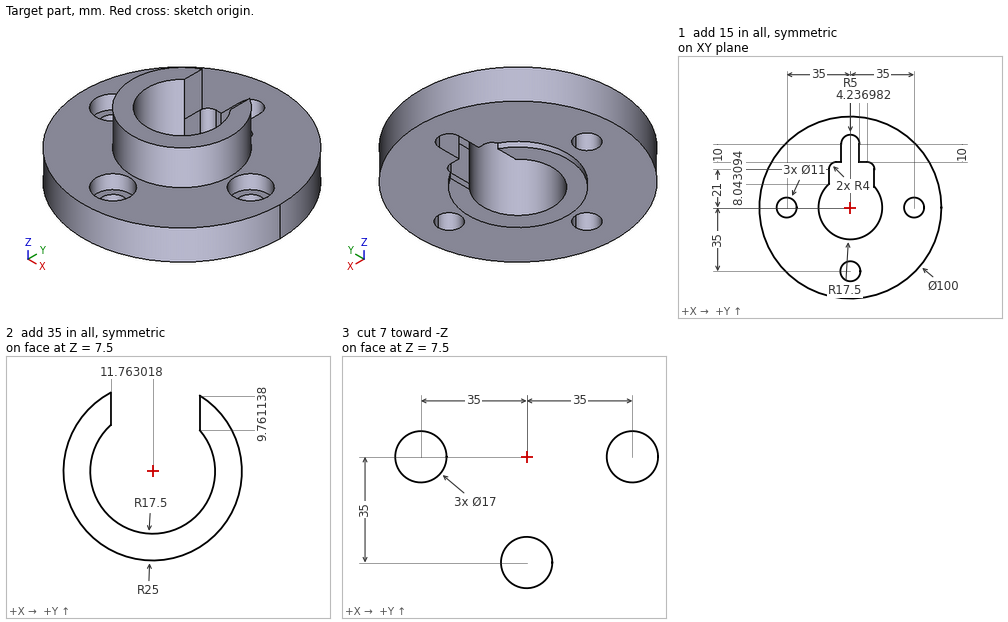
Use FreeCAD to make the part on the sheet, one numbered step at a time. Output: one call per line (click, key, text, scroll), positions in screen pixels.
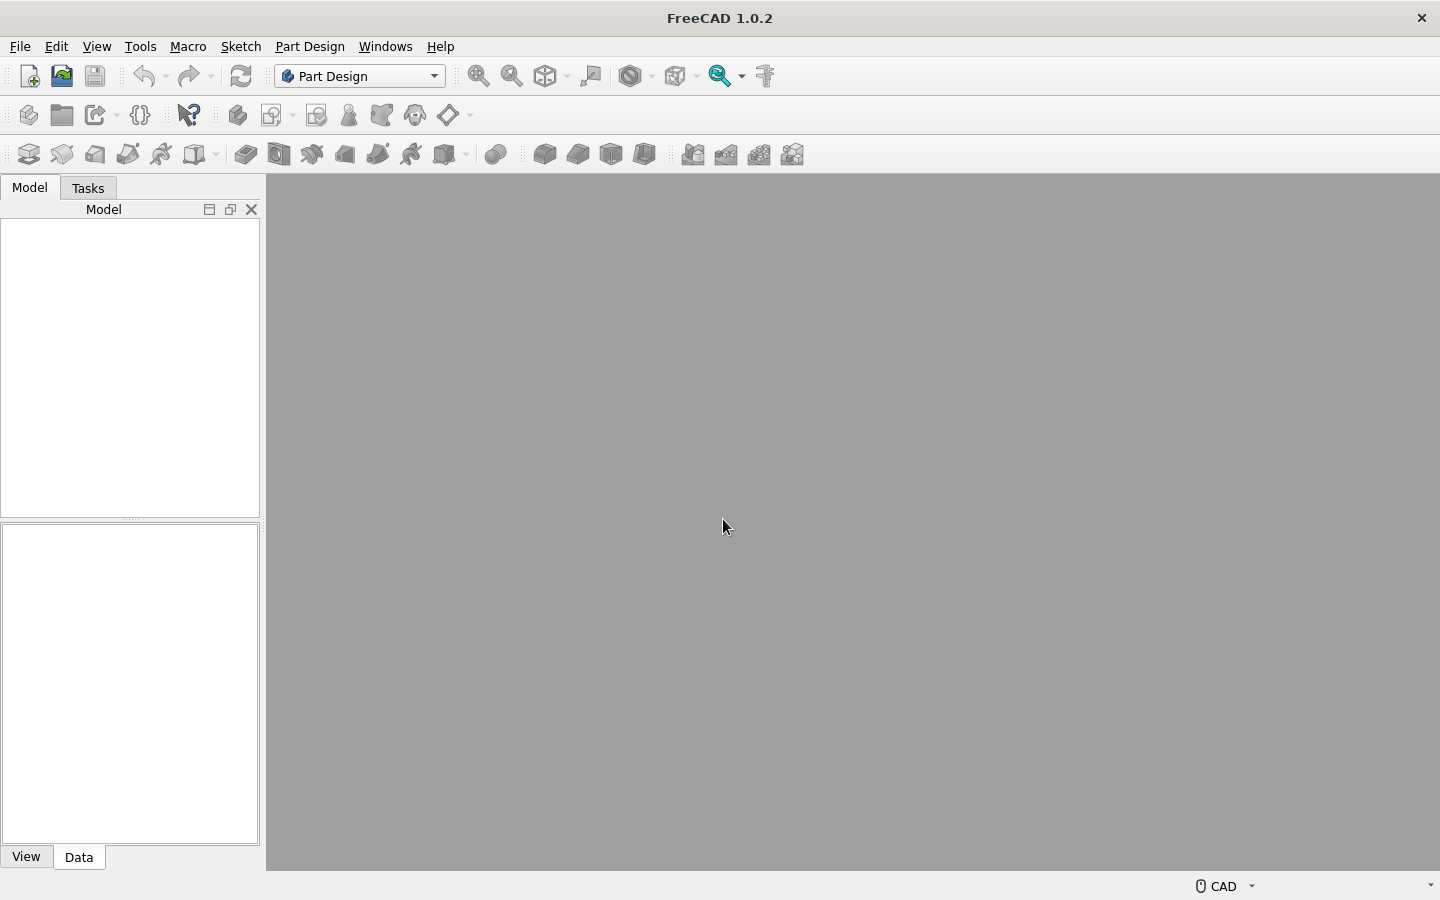
click(29, 76)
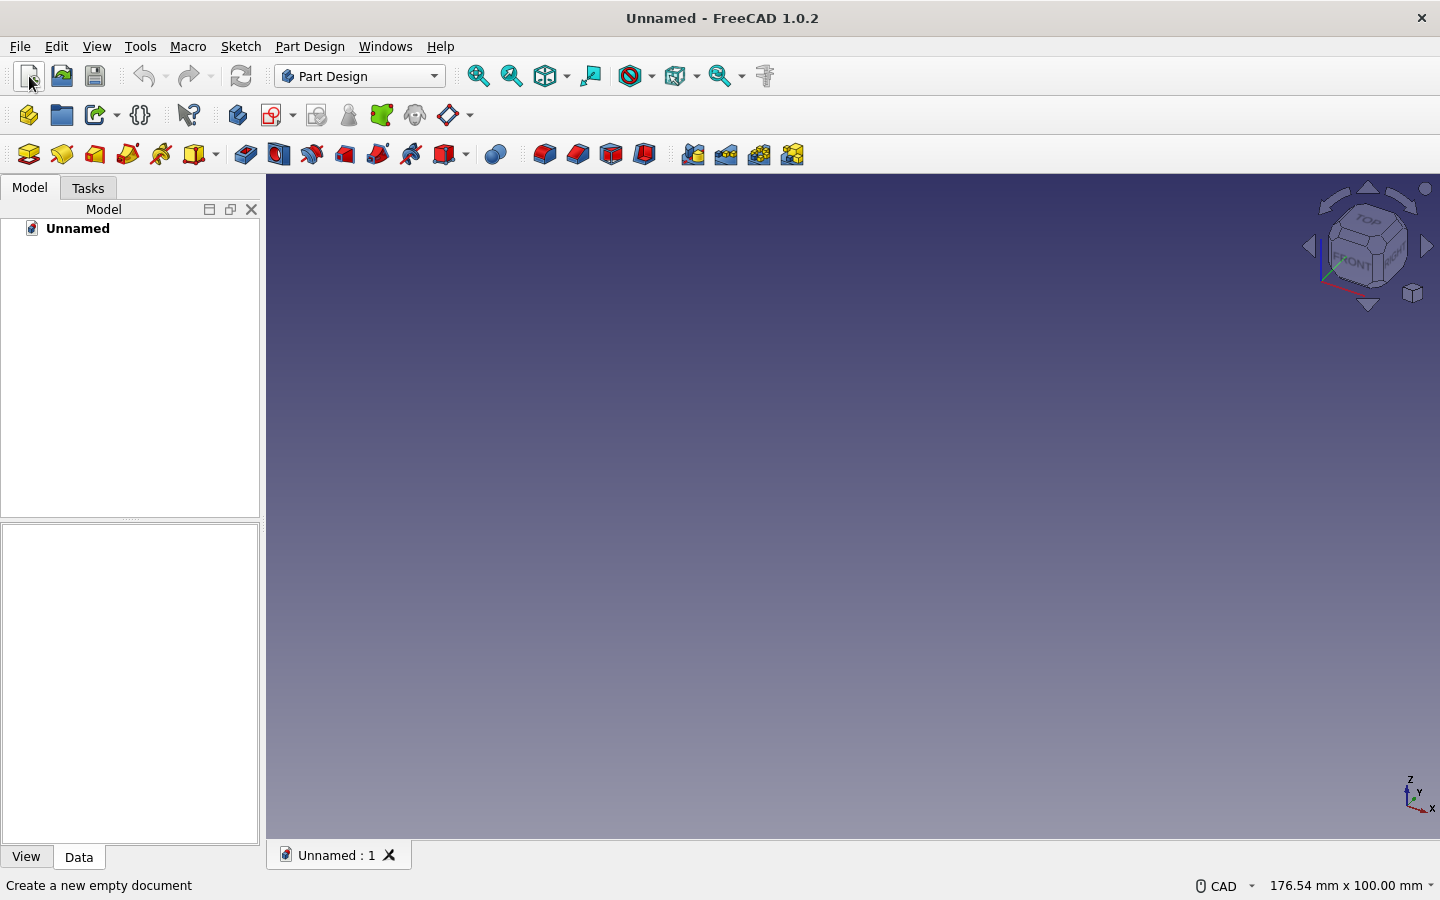
click(270, 116)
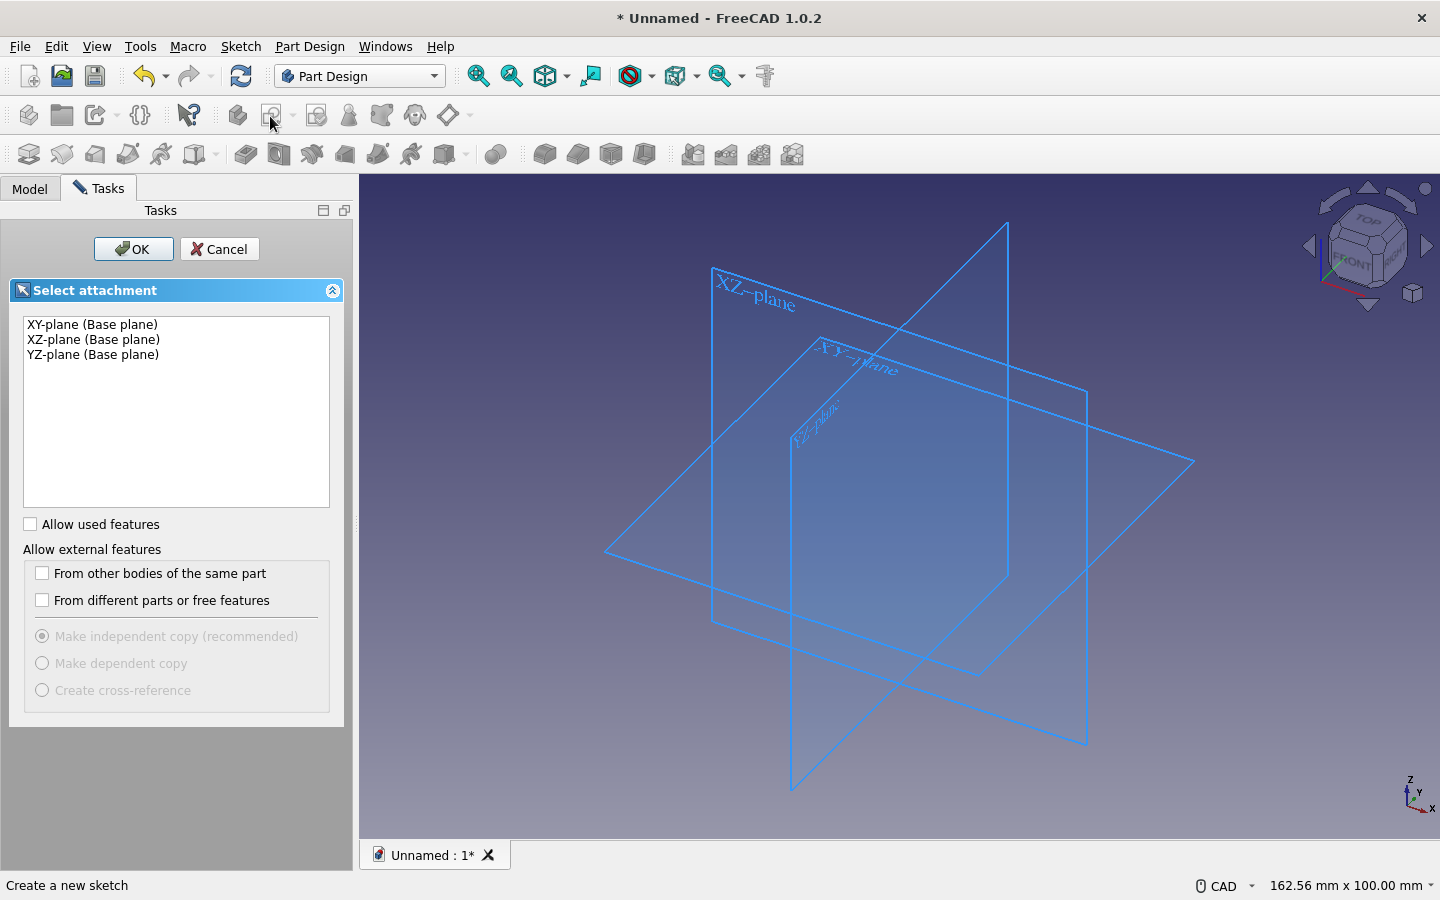
click(84, 324)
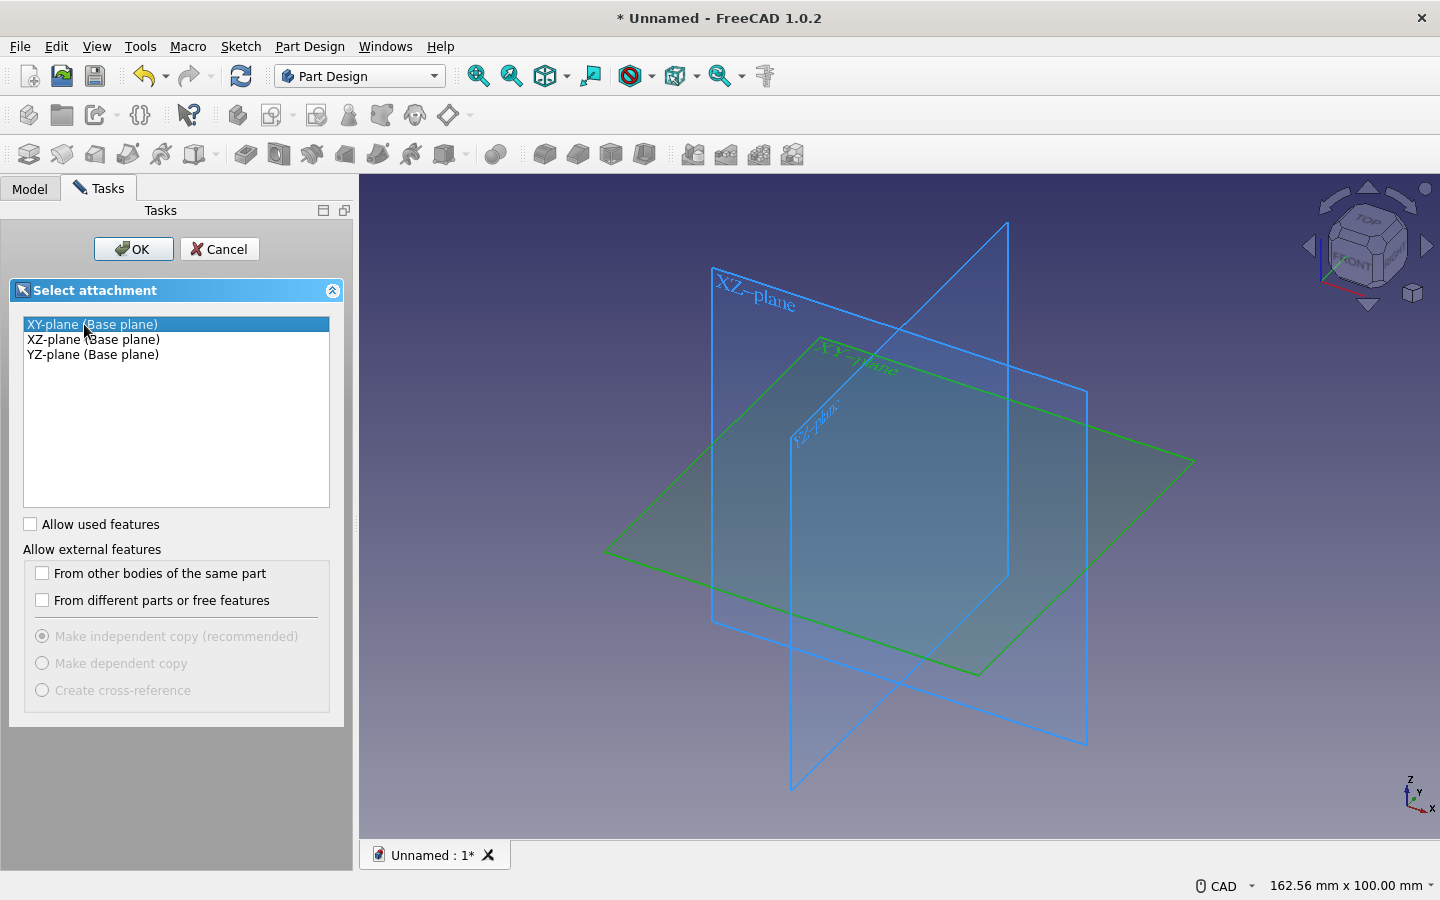
click(134, 249)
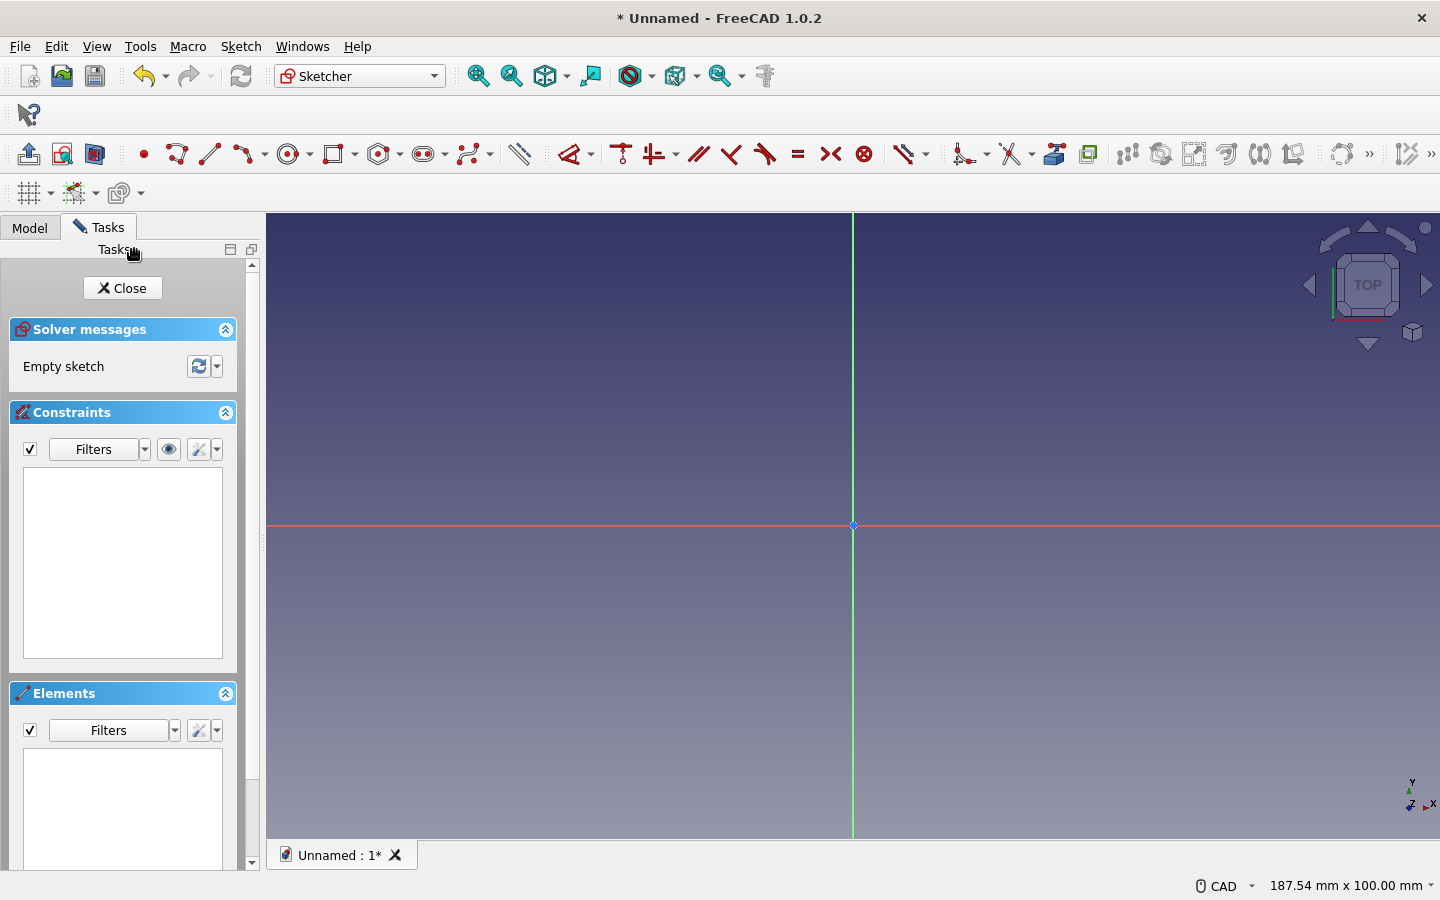
scroll(645, 526, down, 2)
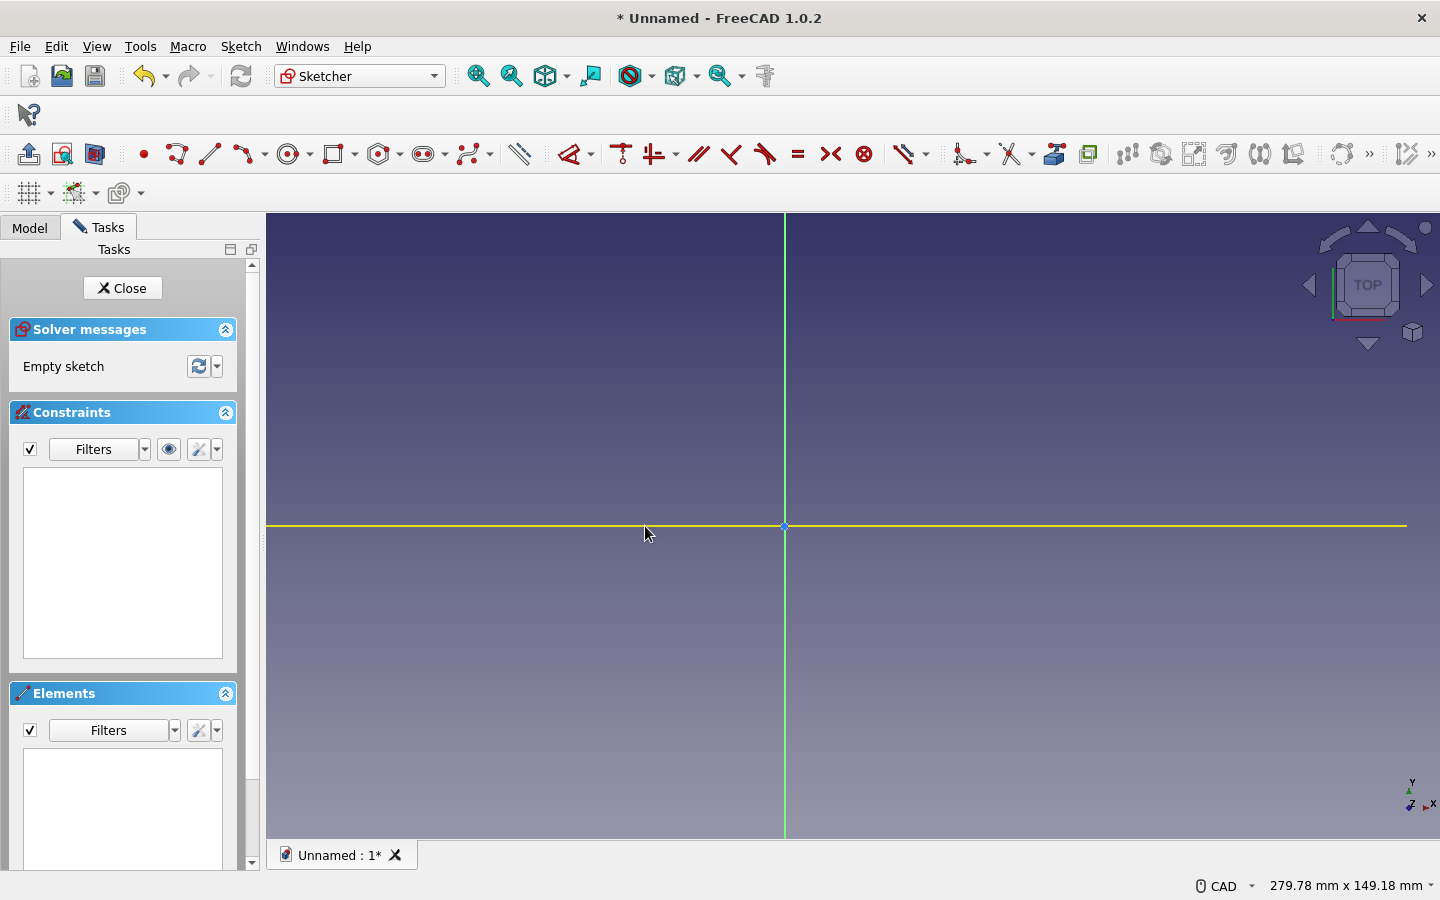
click(210, 154)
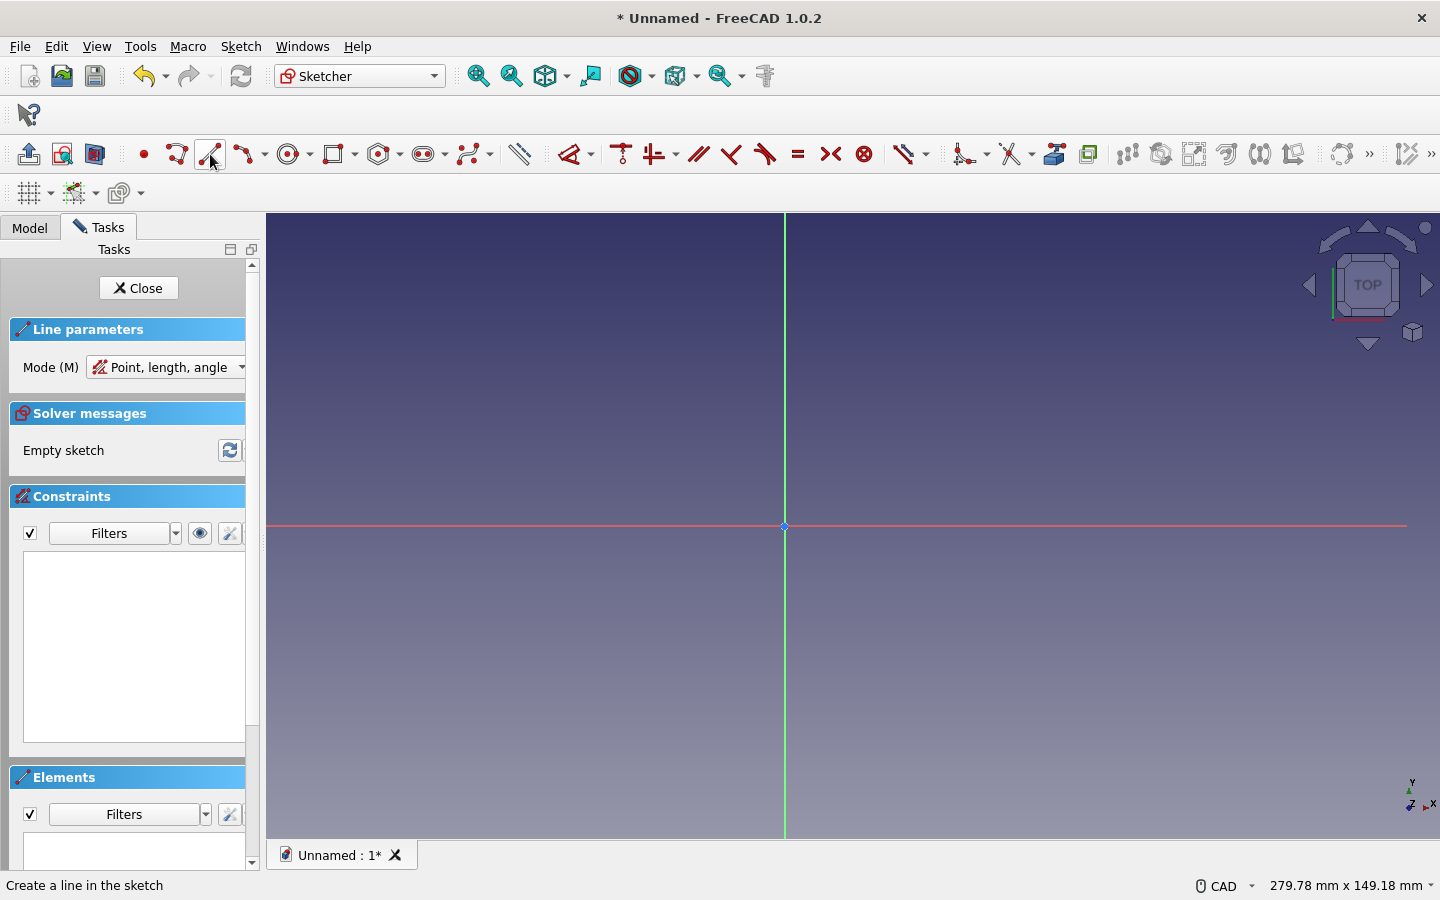
click(735, 472)
click(735, 438)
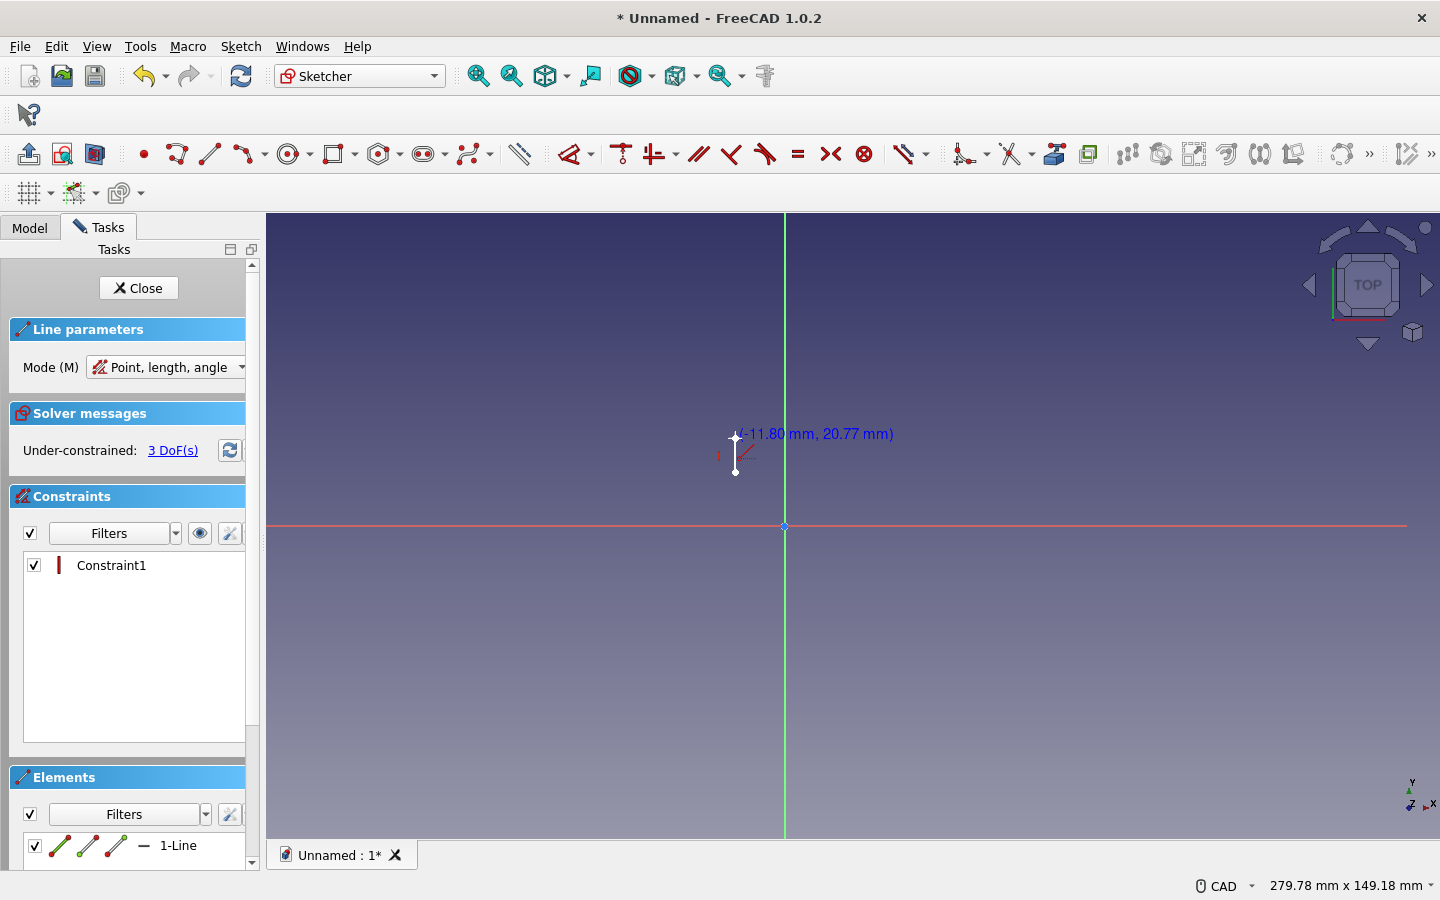
click(177, 154)